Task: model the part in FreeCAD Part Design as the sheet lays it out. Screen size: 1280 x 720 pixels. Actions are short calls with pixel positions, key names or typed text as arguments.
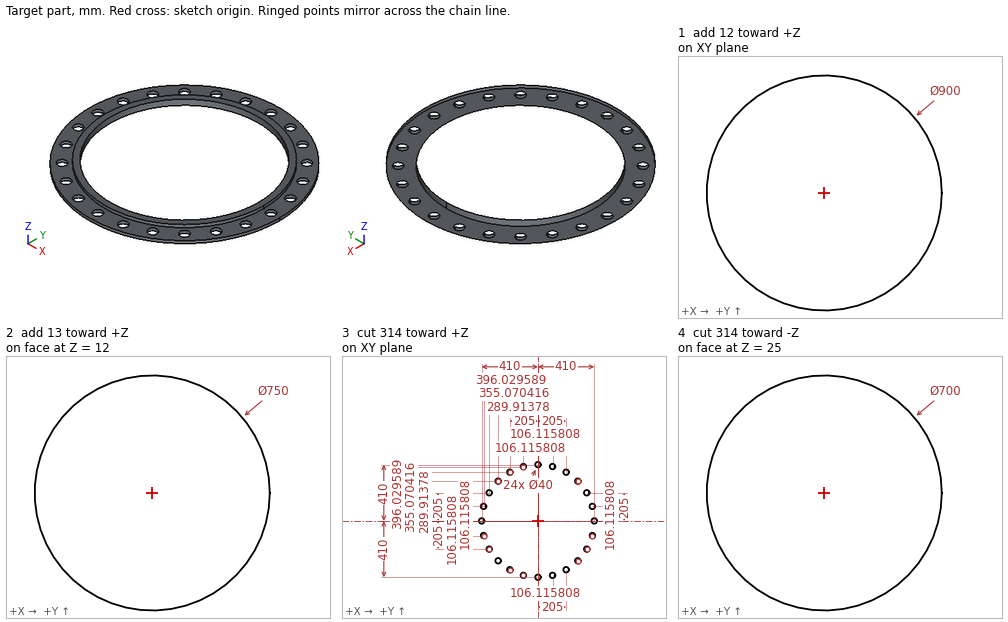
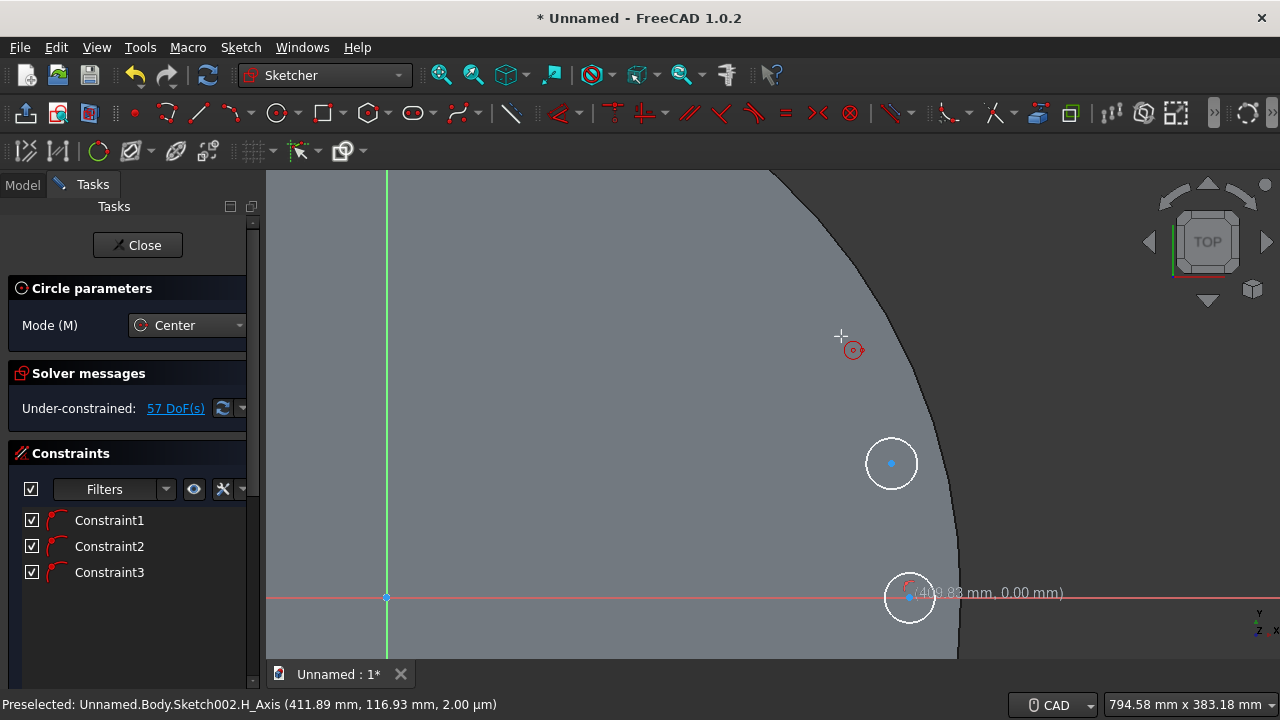
click(840, 336)
click(858, 318)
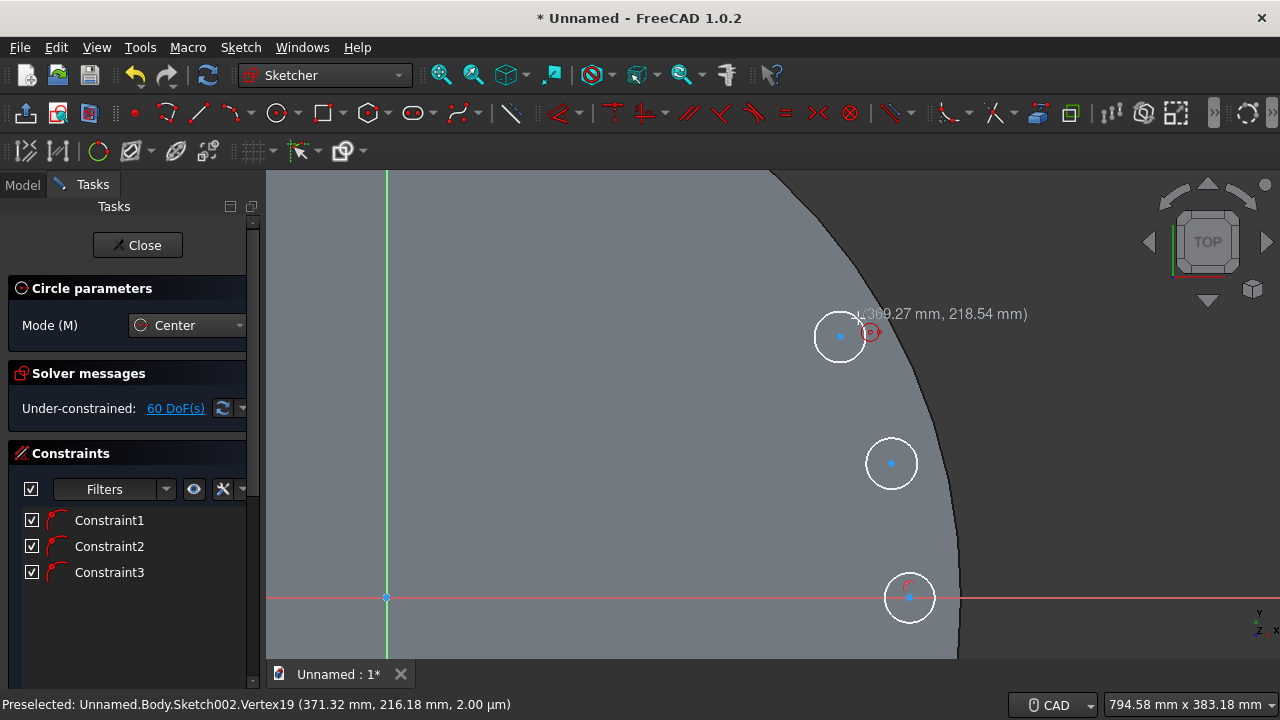
click(757, 228)
click(775, 210)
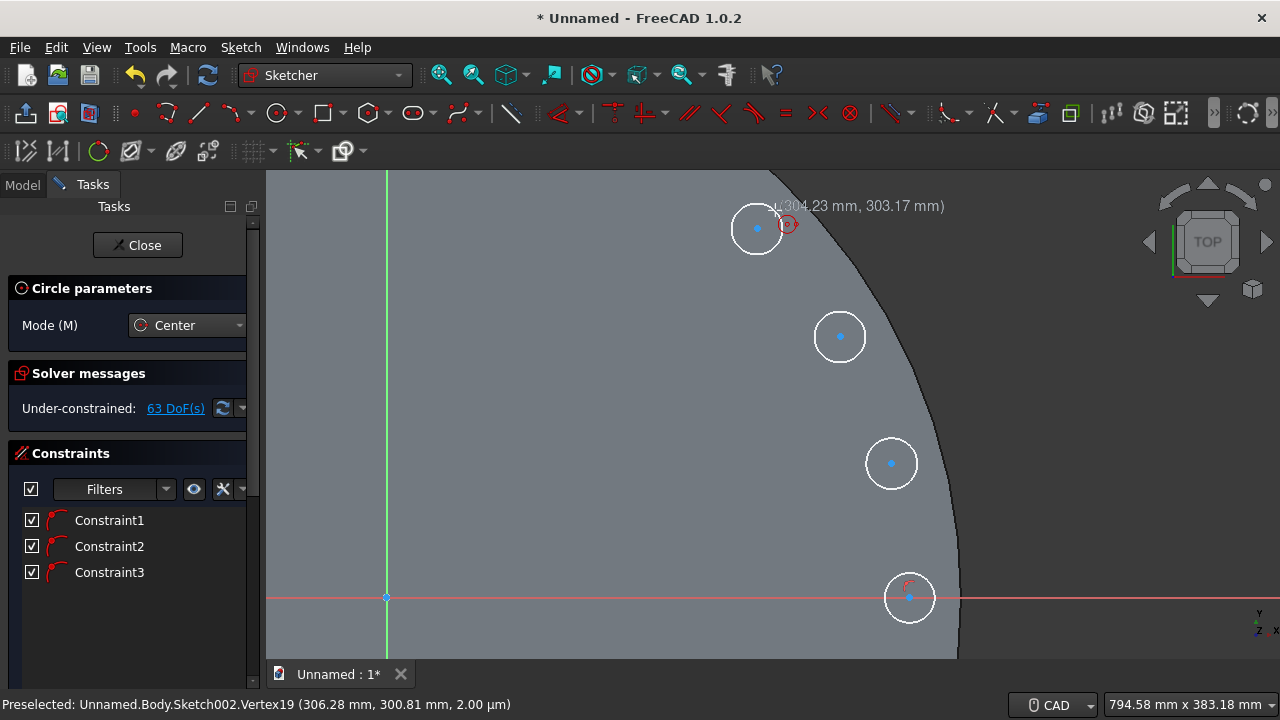
scroll(841, 335, down, 6)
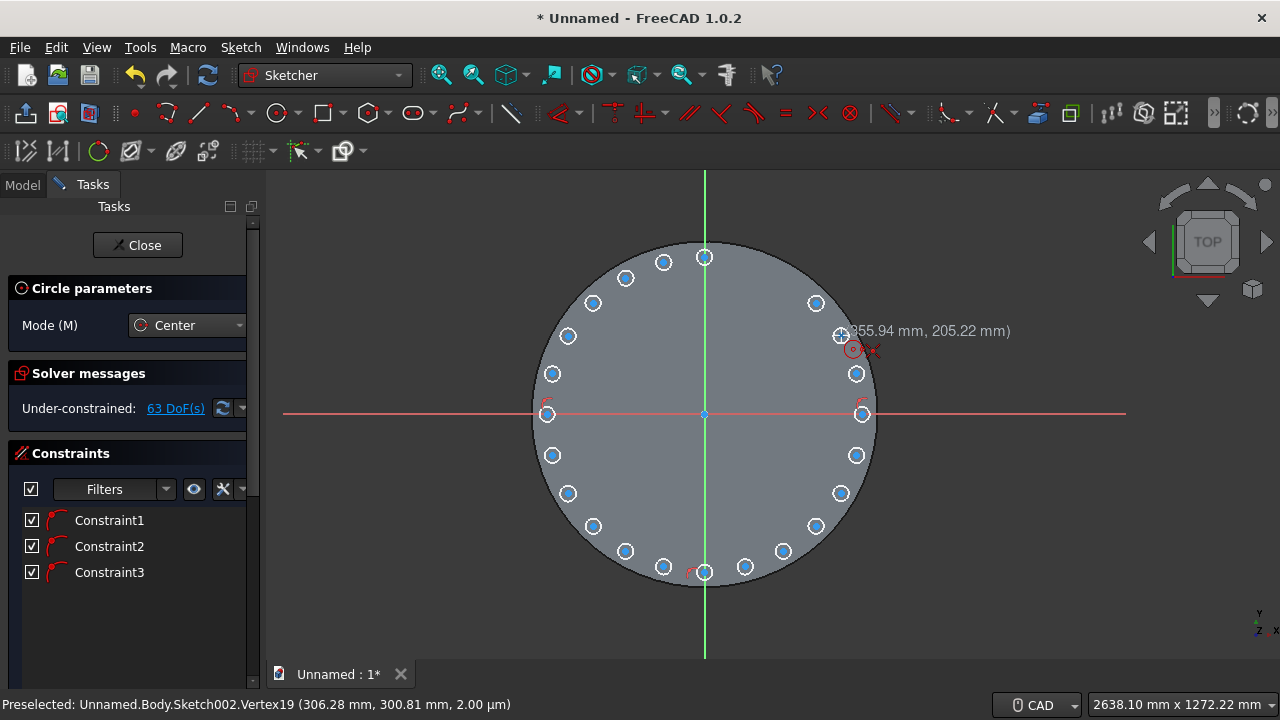
scroll(783, 278, up, 6)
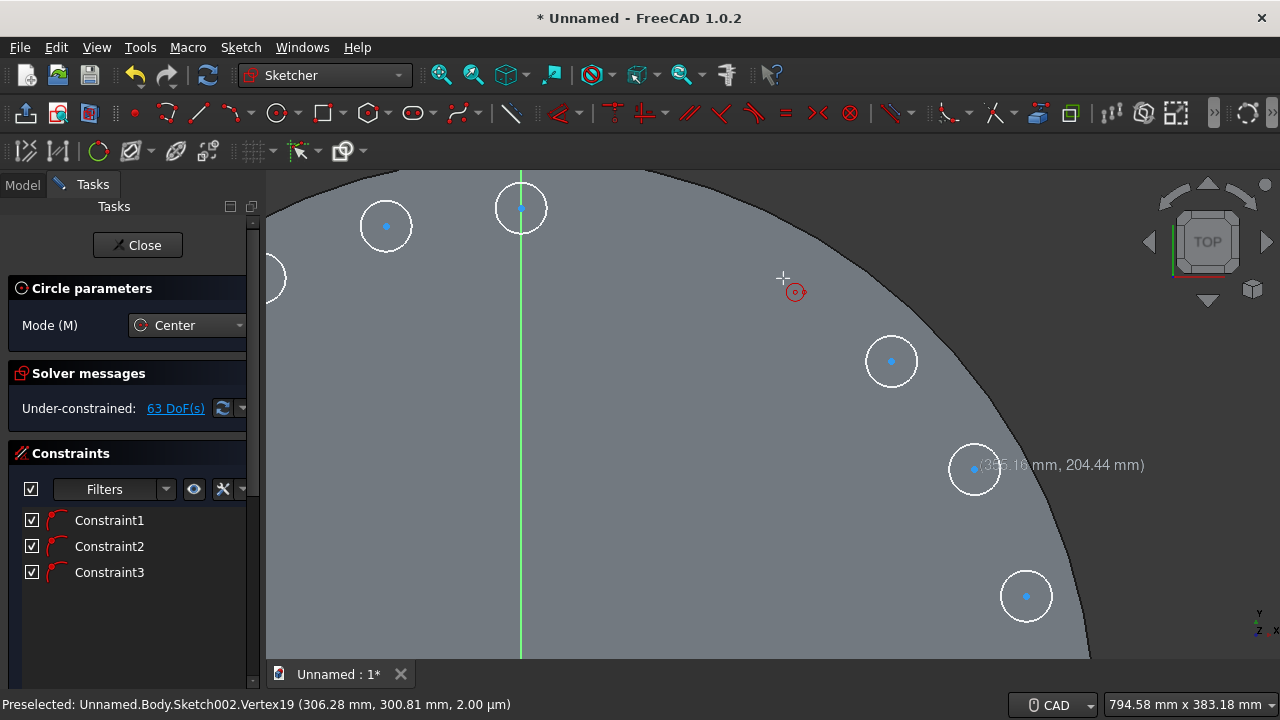
click(783, 277)
click(801, 259)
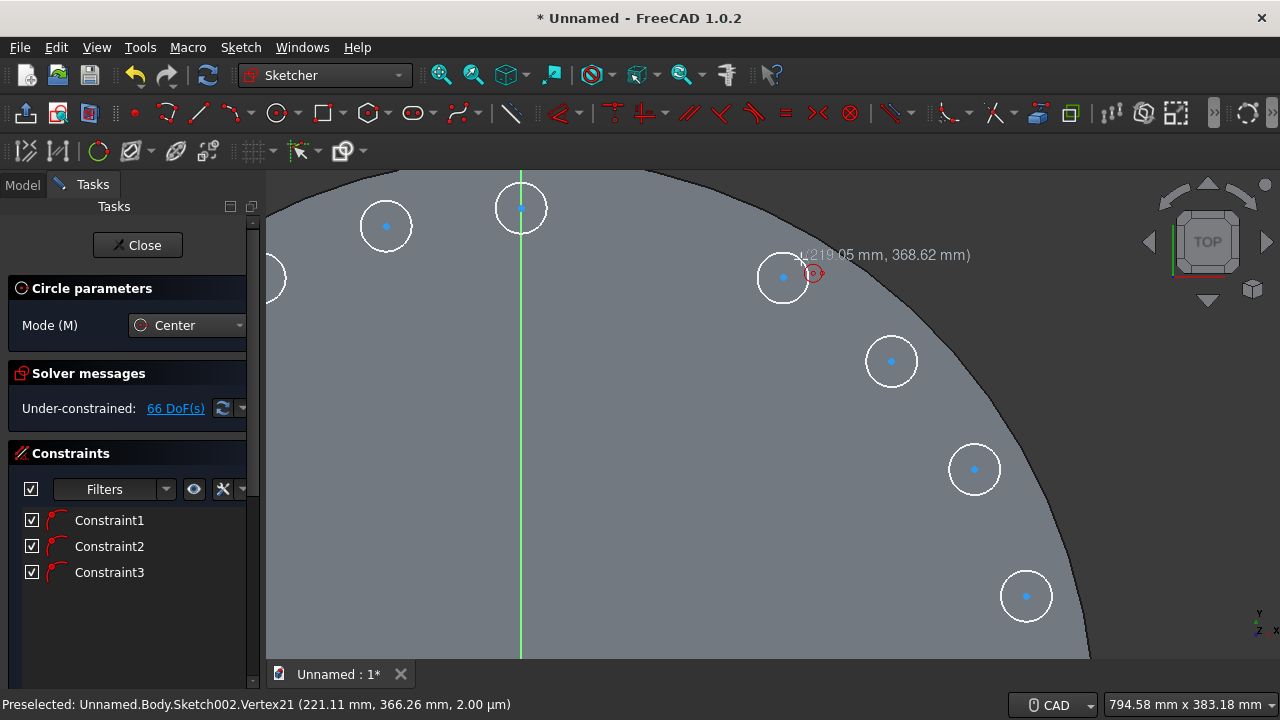
click(657, 225)
click(675, 207)
key(Escape)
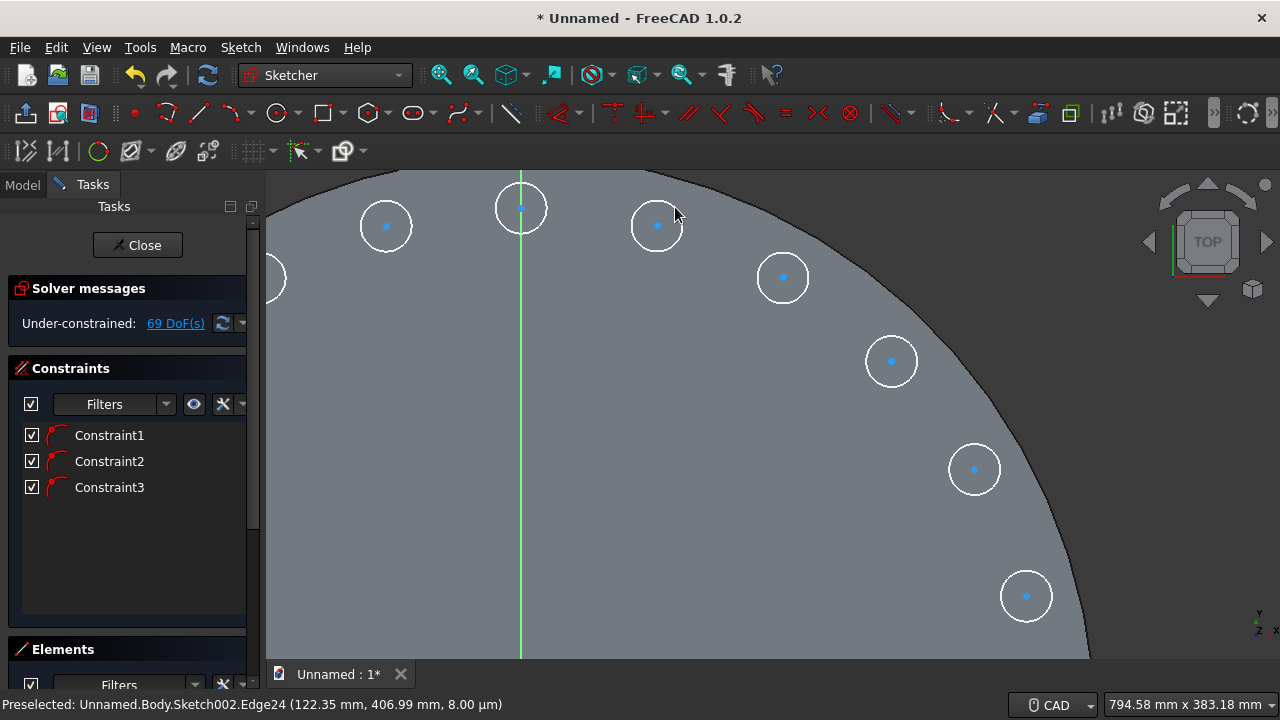
click(503, 226)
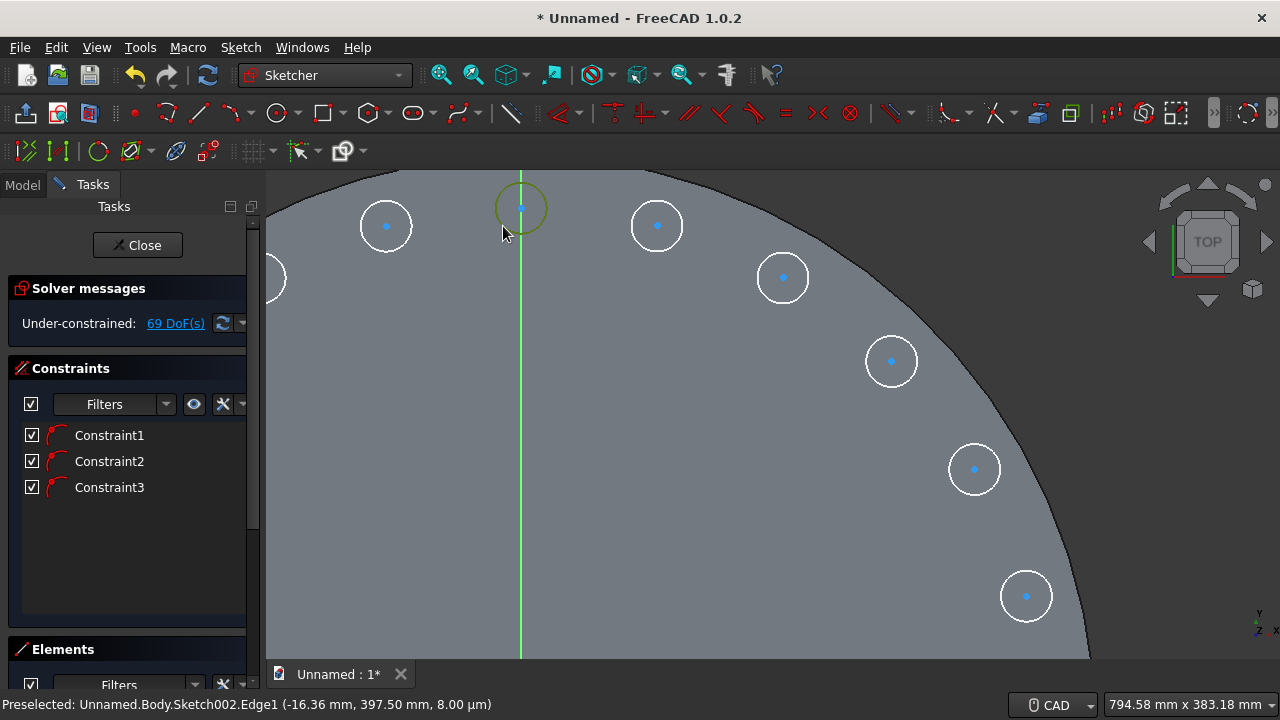
click(404, 208)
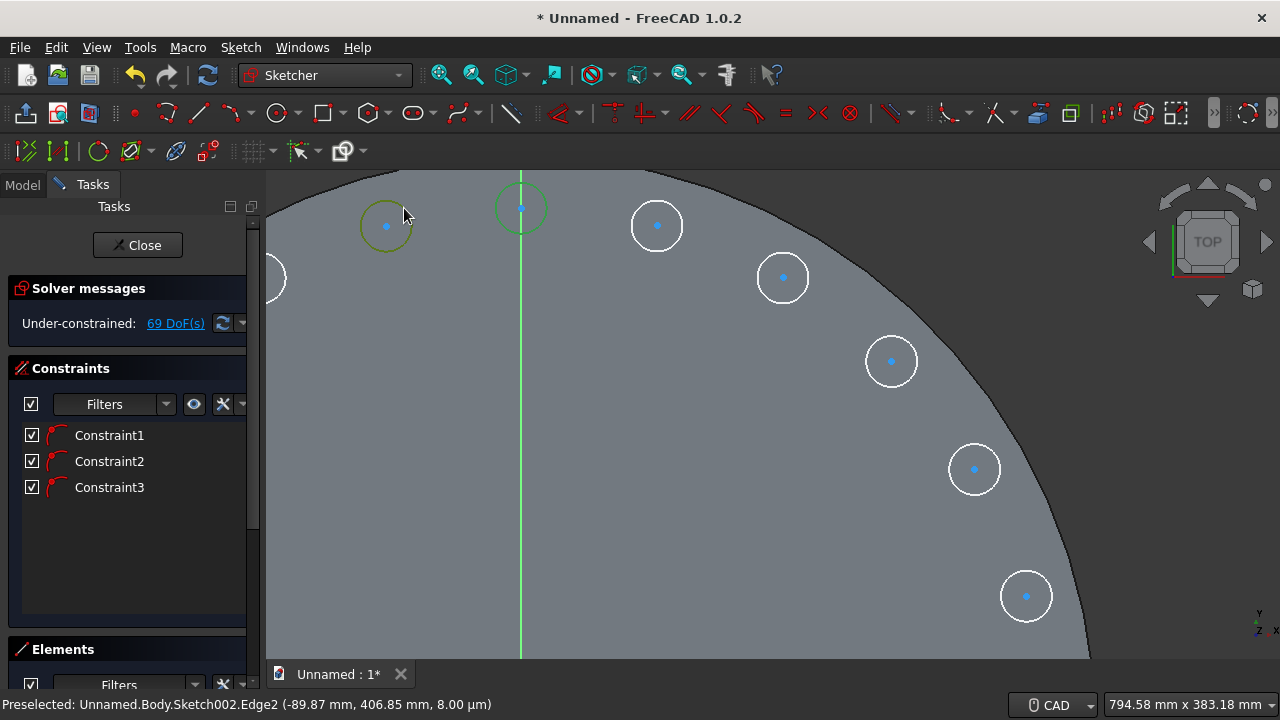
scroll(783, 278, down, 6)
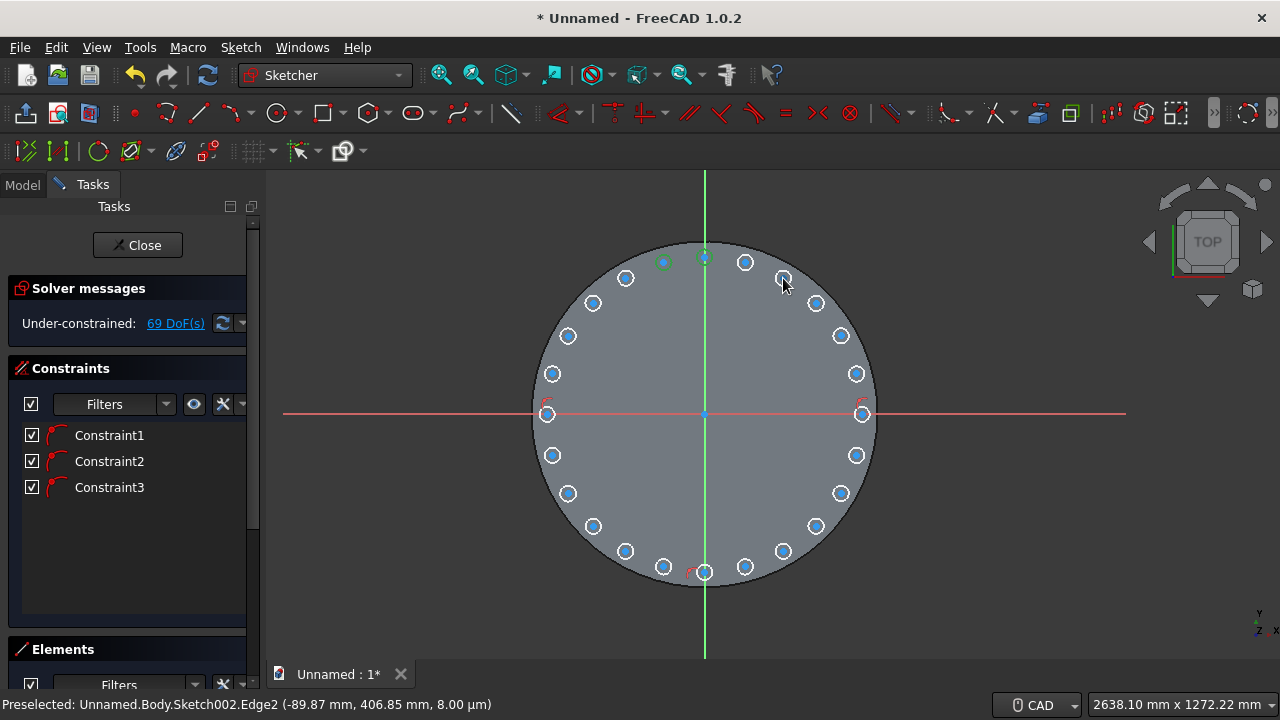
scroll(631, 273, up, 3)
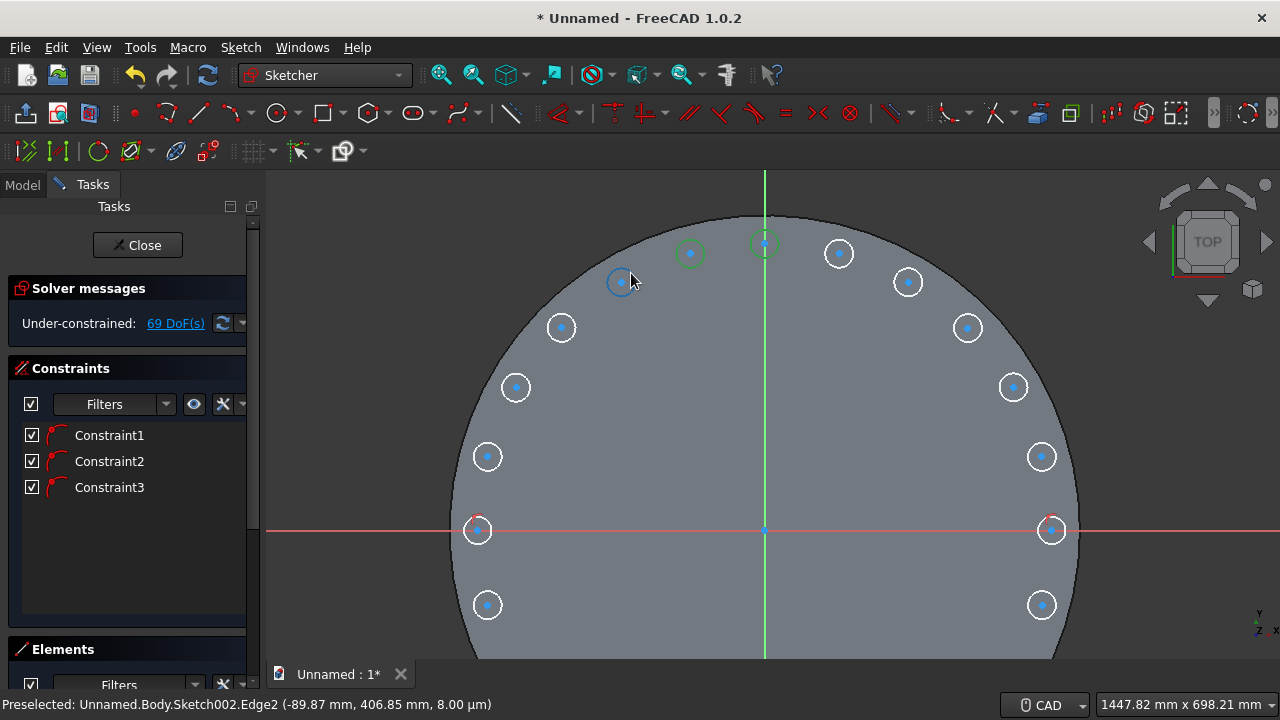
click(631, 272)